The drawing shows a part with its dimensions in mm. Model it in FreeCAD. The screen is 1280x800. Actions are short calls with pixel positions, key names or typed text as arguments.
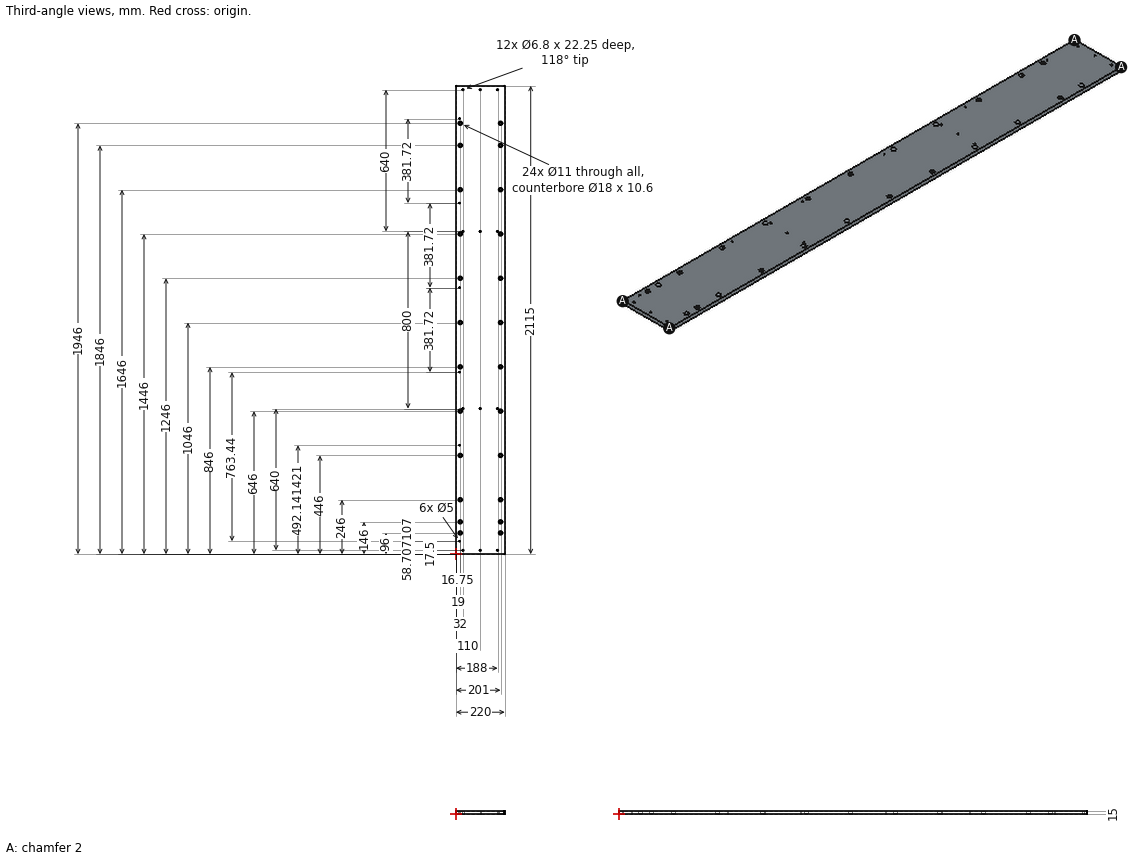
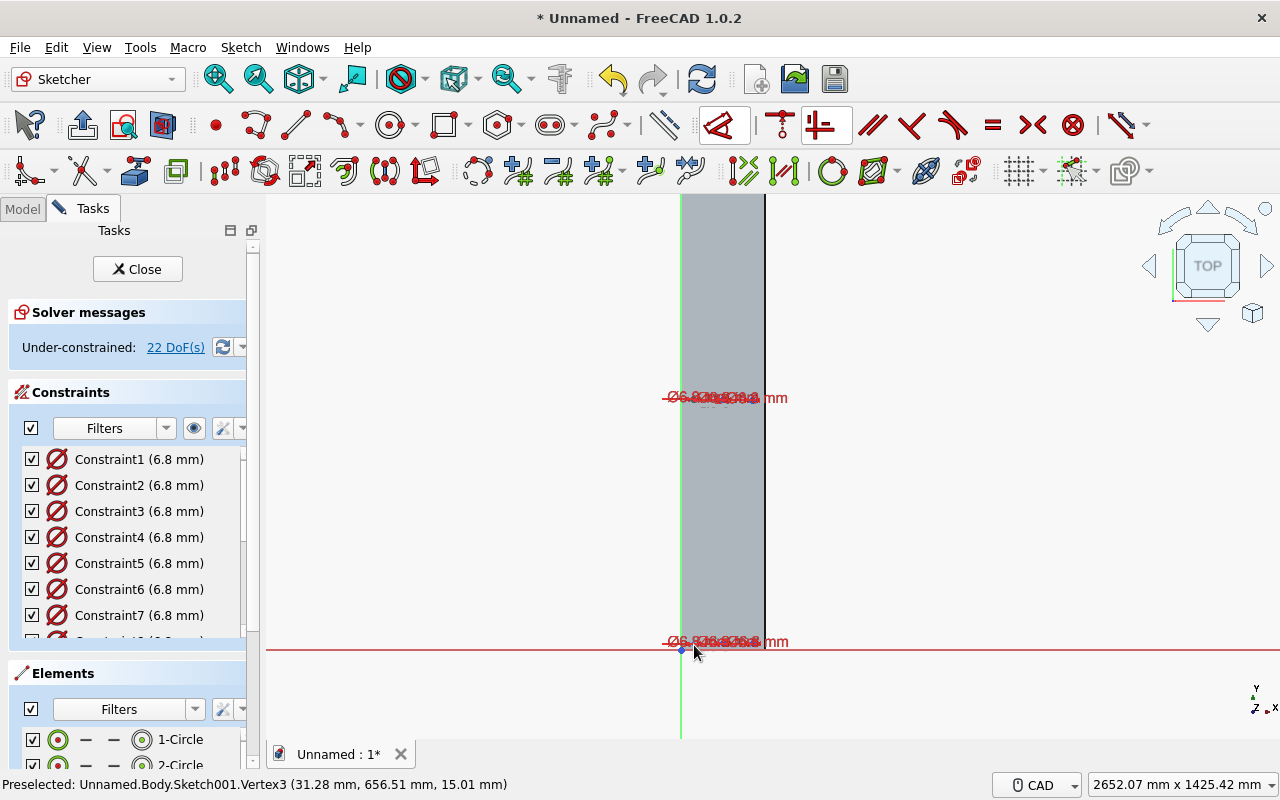
click(693, 644)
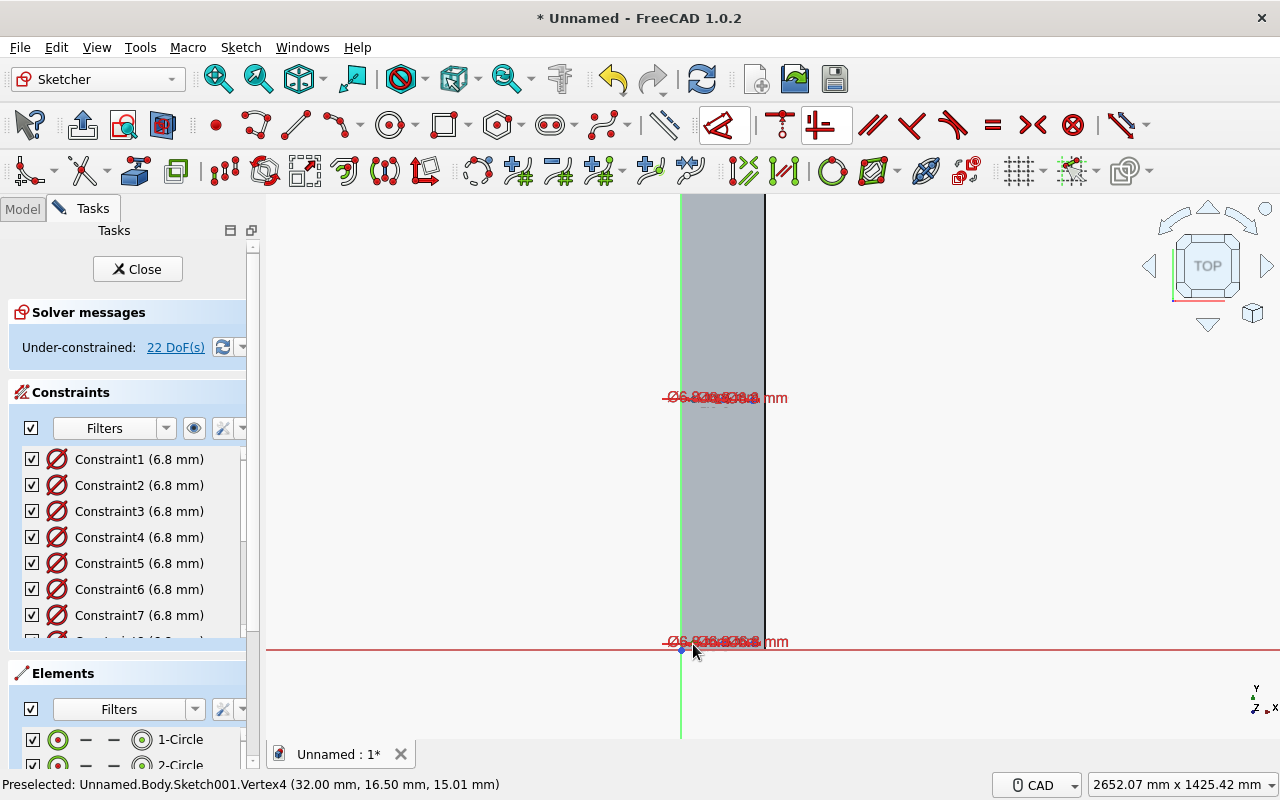
click(846, 126)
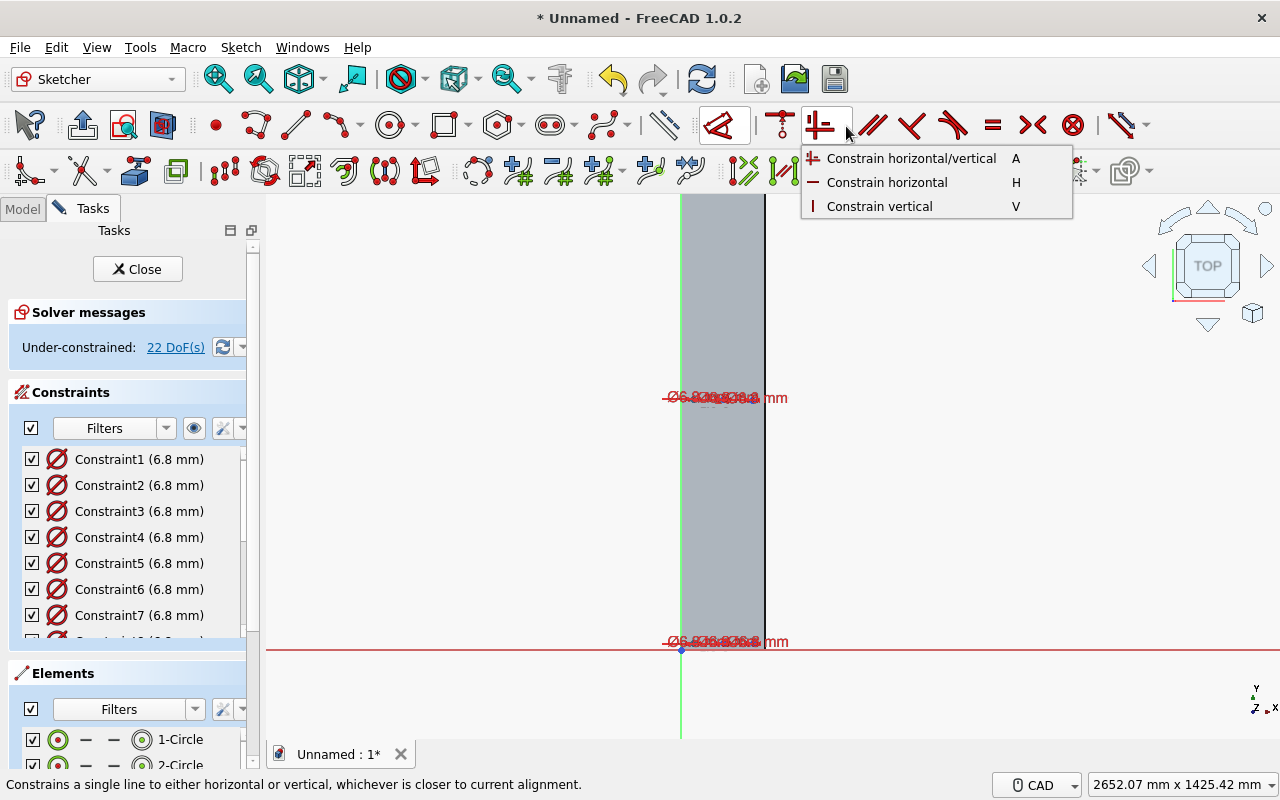
click(937, 206)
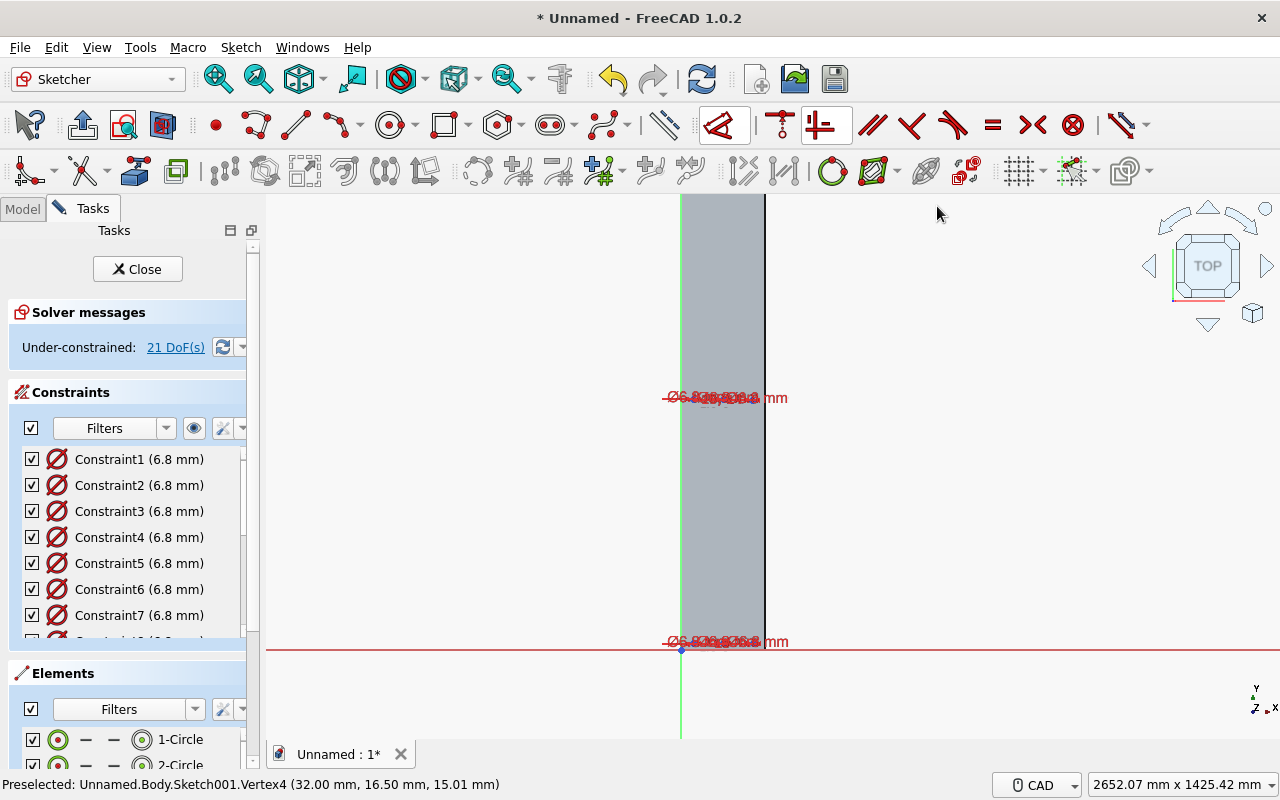
scroll(694, 644, down, 4)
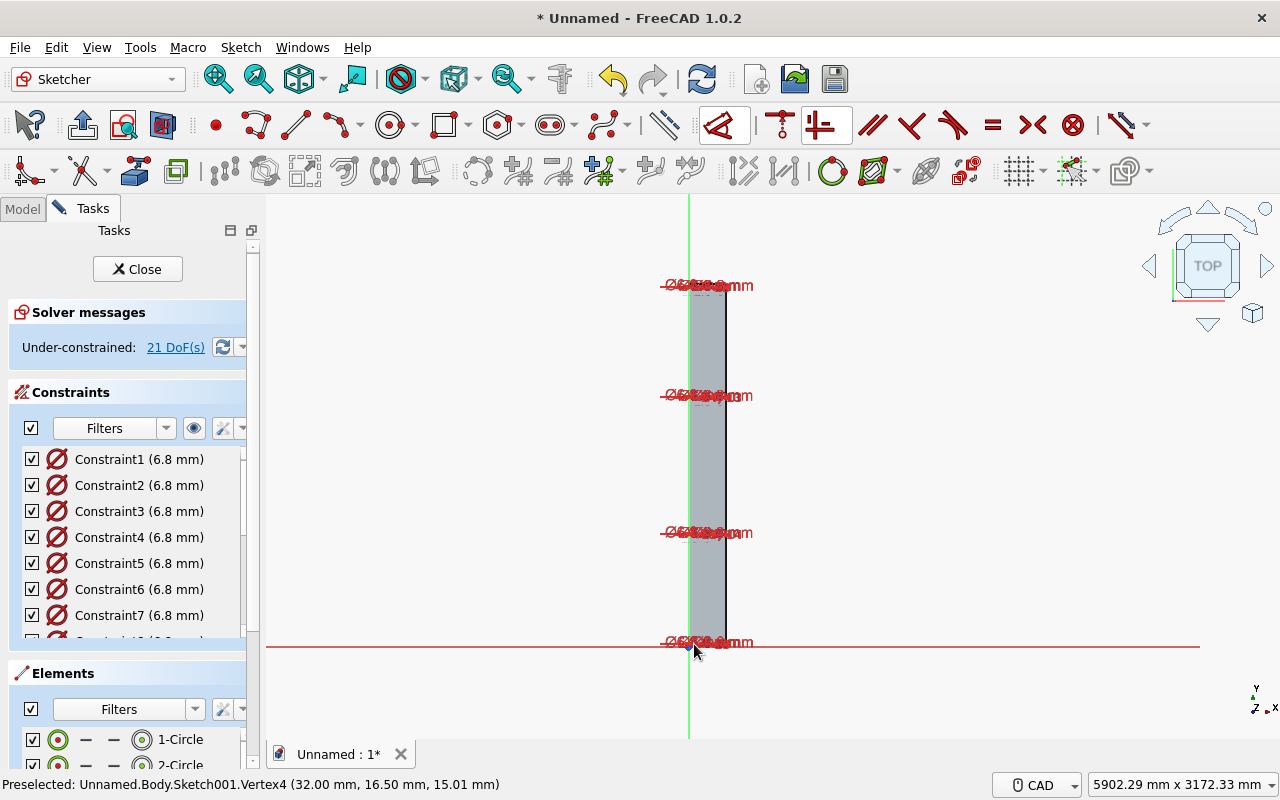
click(694, 287)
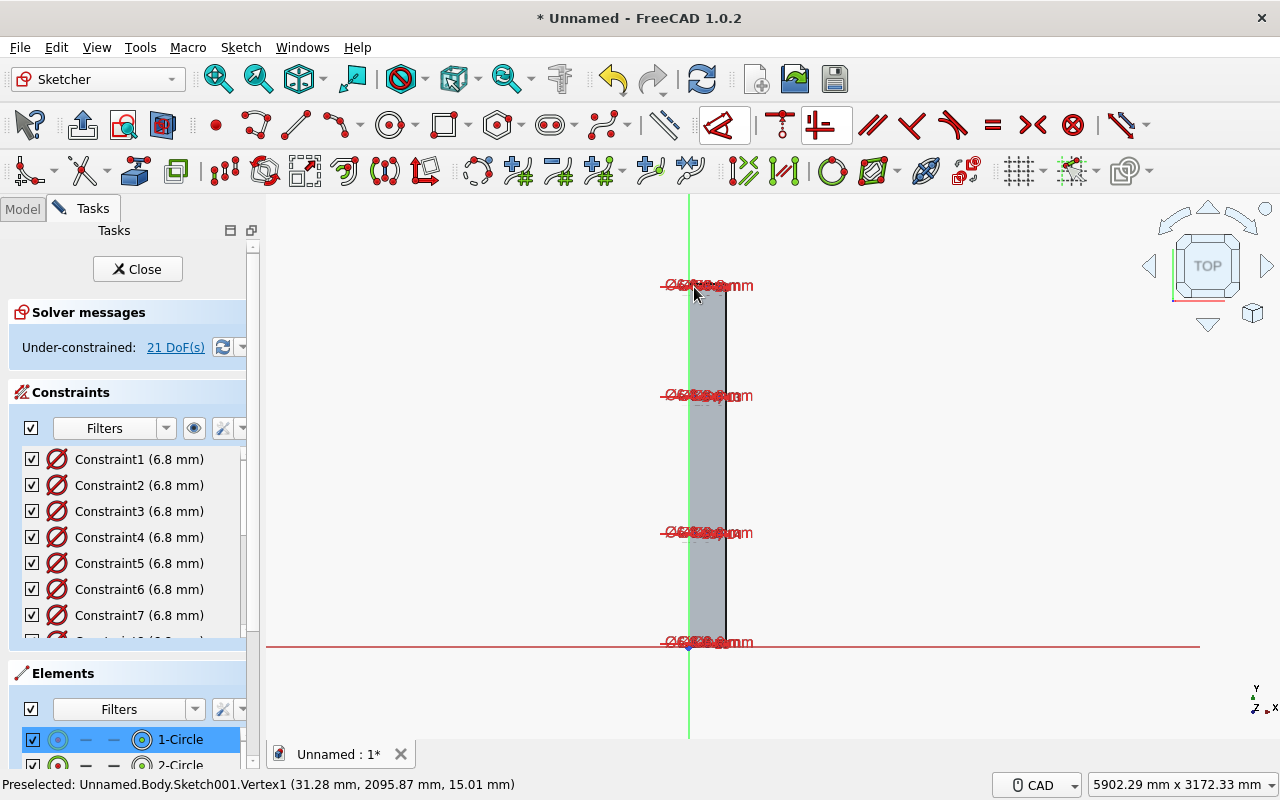
click(708, 288)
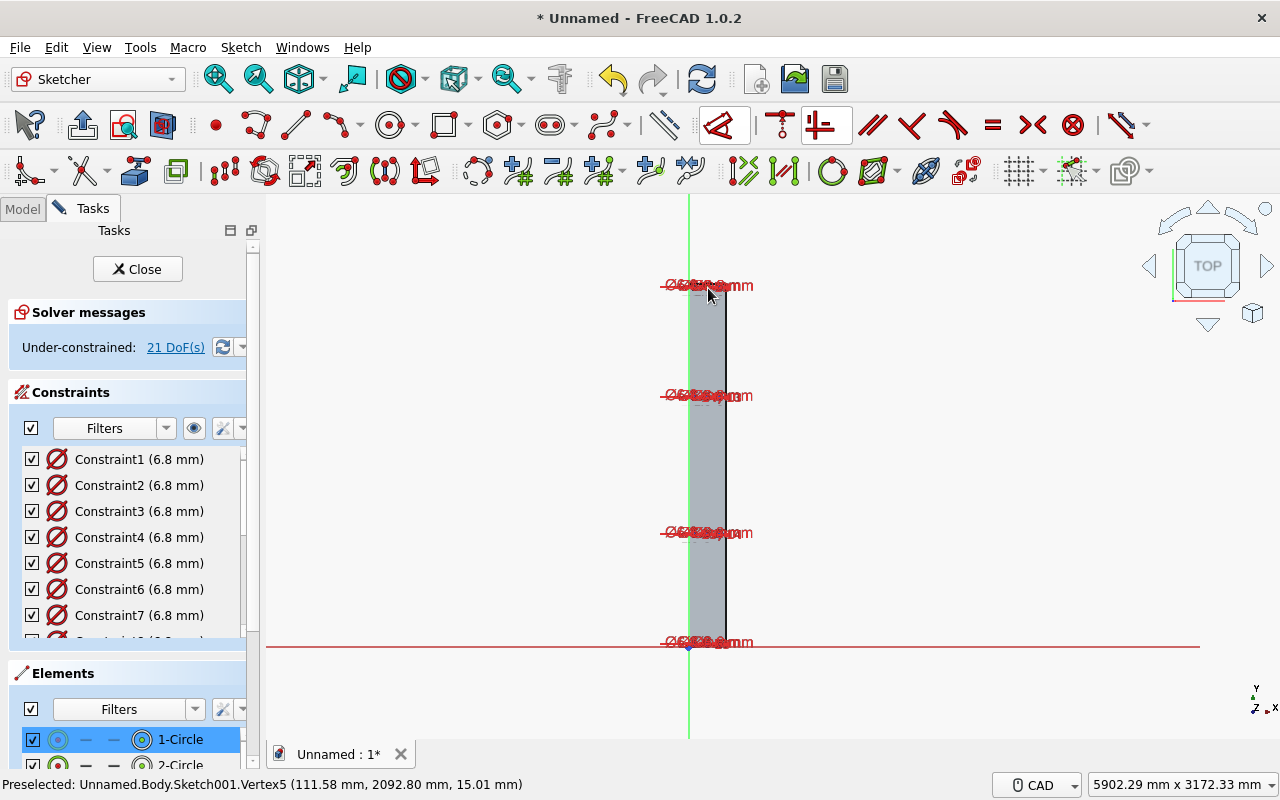
click(846, 126)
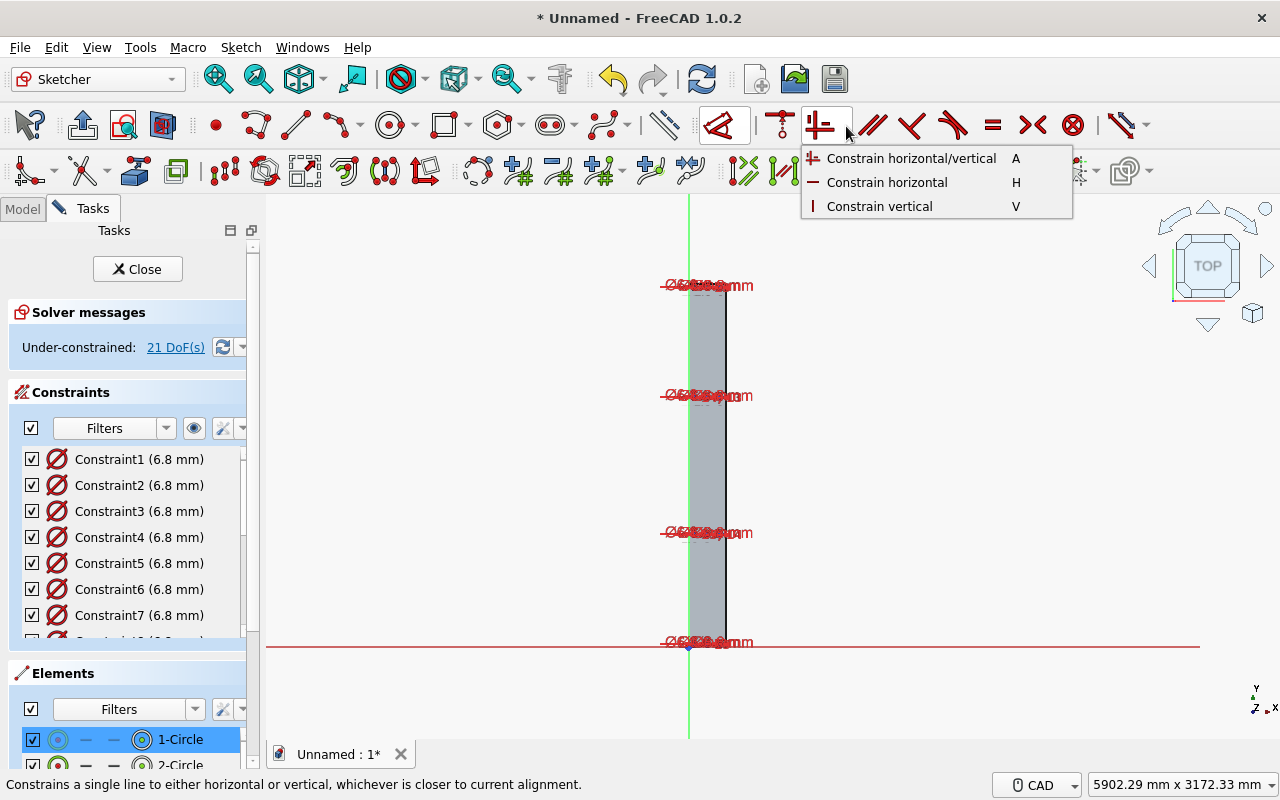
click(937, 182)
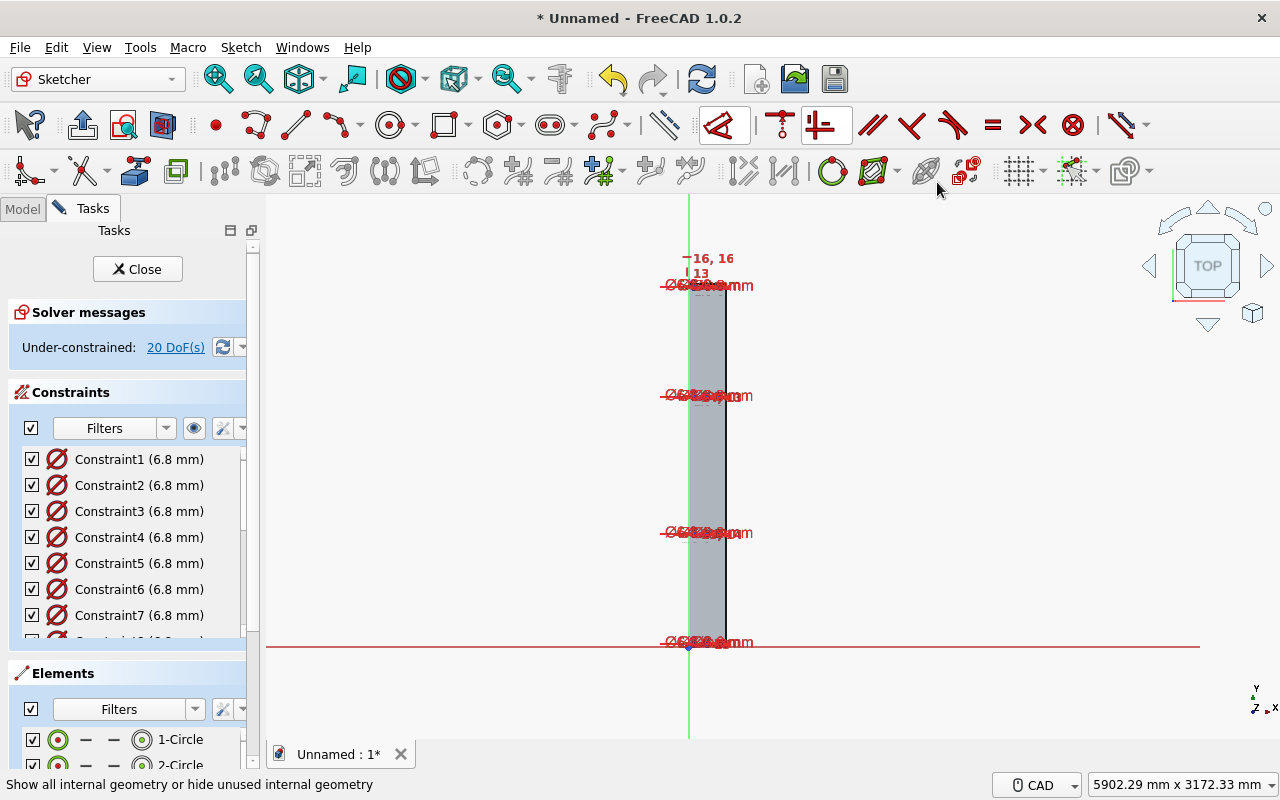
click(708, 287)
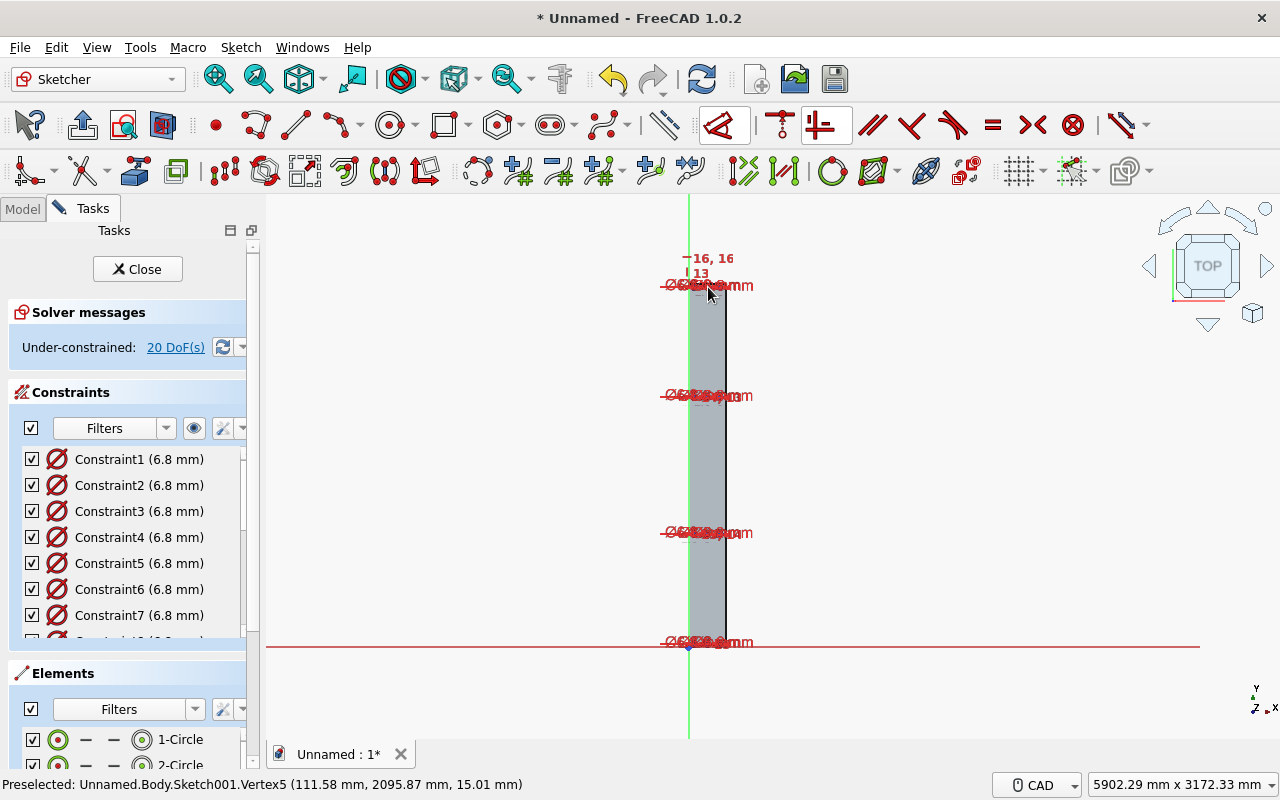
click(707, 398)